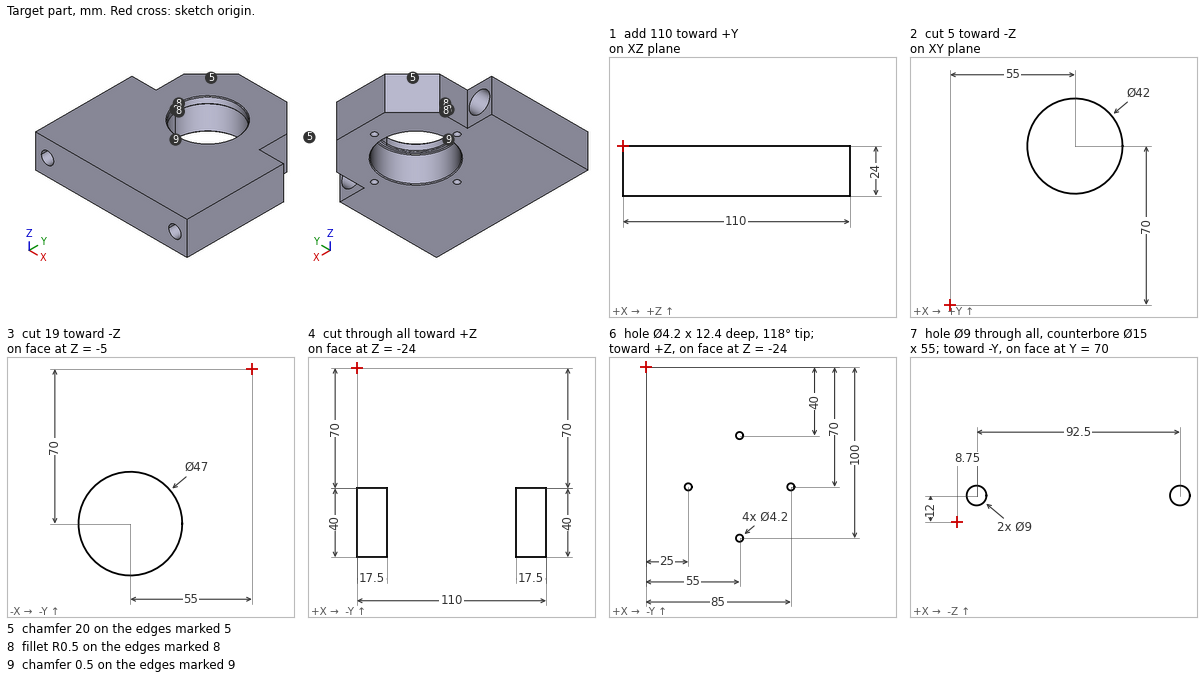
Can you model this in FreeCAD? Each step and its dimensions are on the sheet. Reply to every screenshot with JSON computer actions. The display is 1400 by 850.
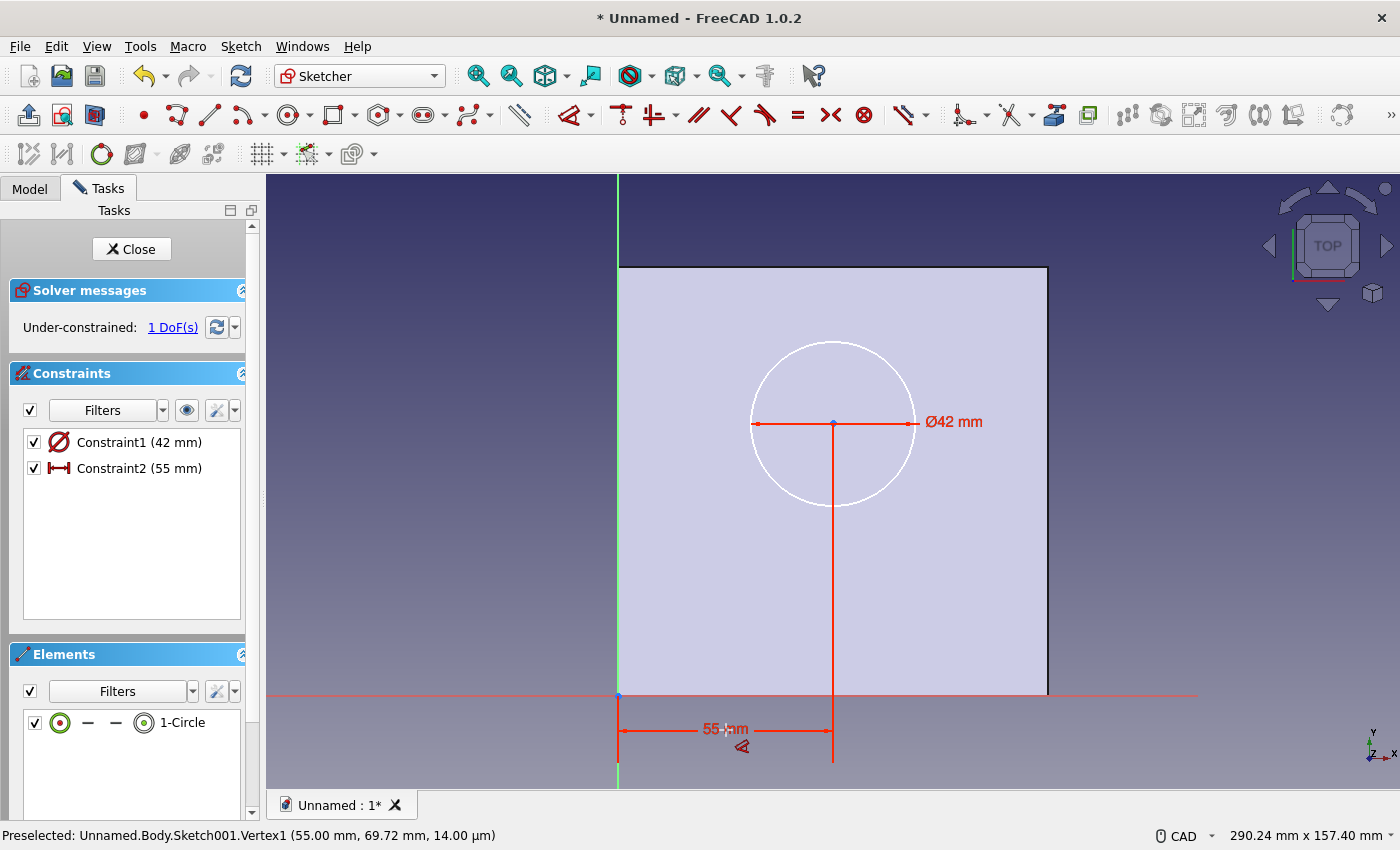
{"action": "left_click", "coordinate": [833, 424]}
{"action": "left_click", "coordinate": [584, 560]}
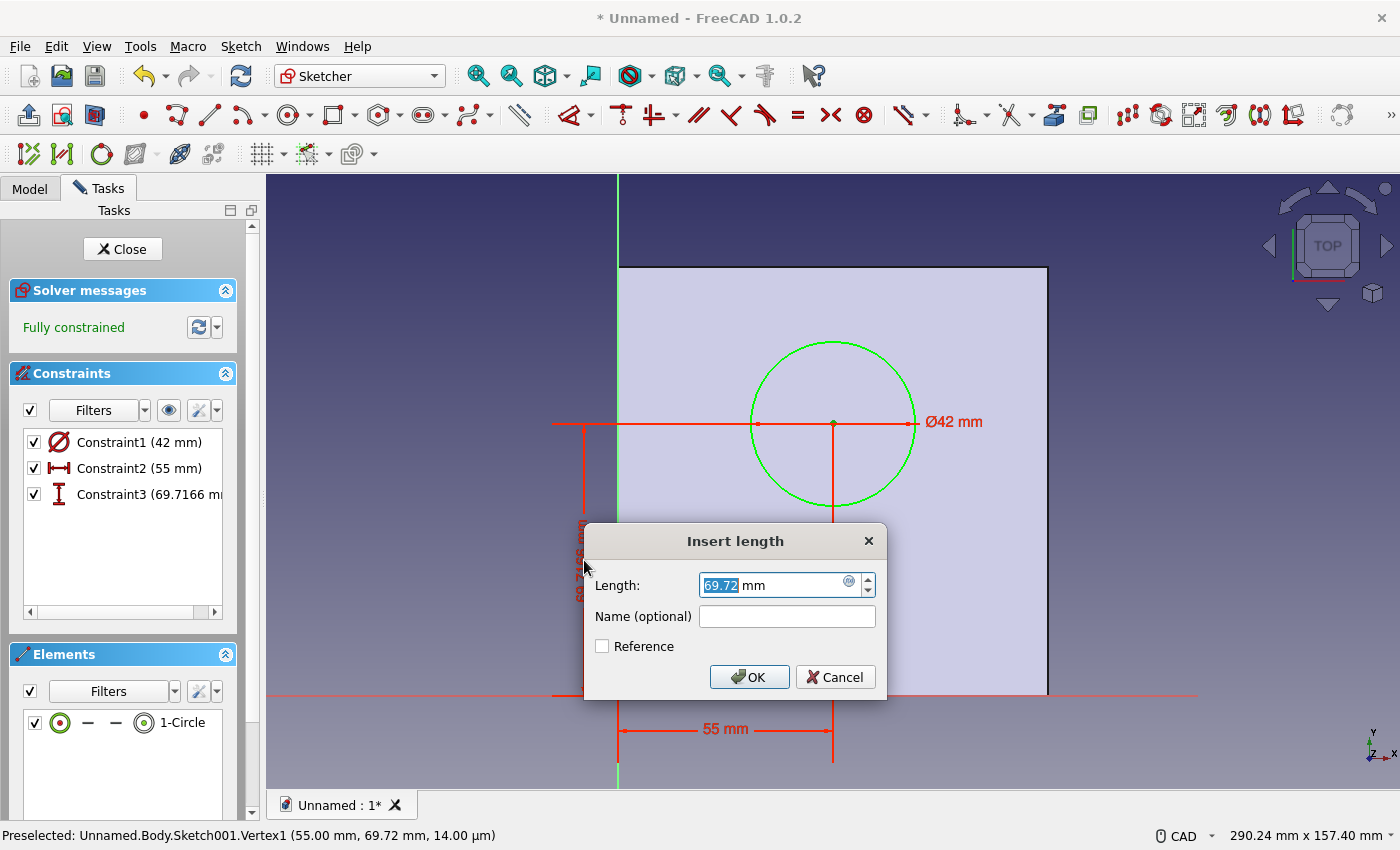
{"action": "type", "text": "70"}
{"action": "key", "text": "Return"}
{"action": "key", "text": "Escape"}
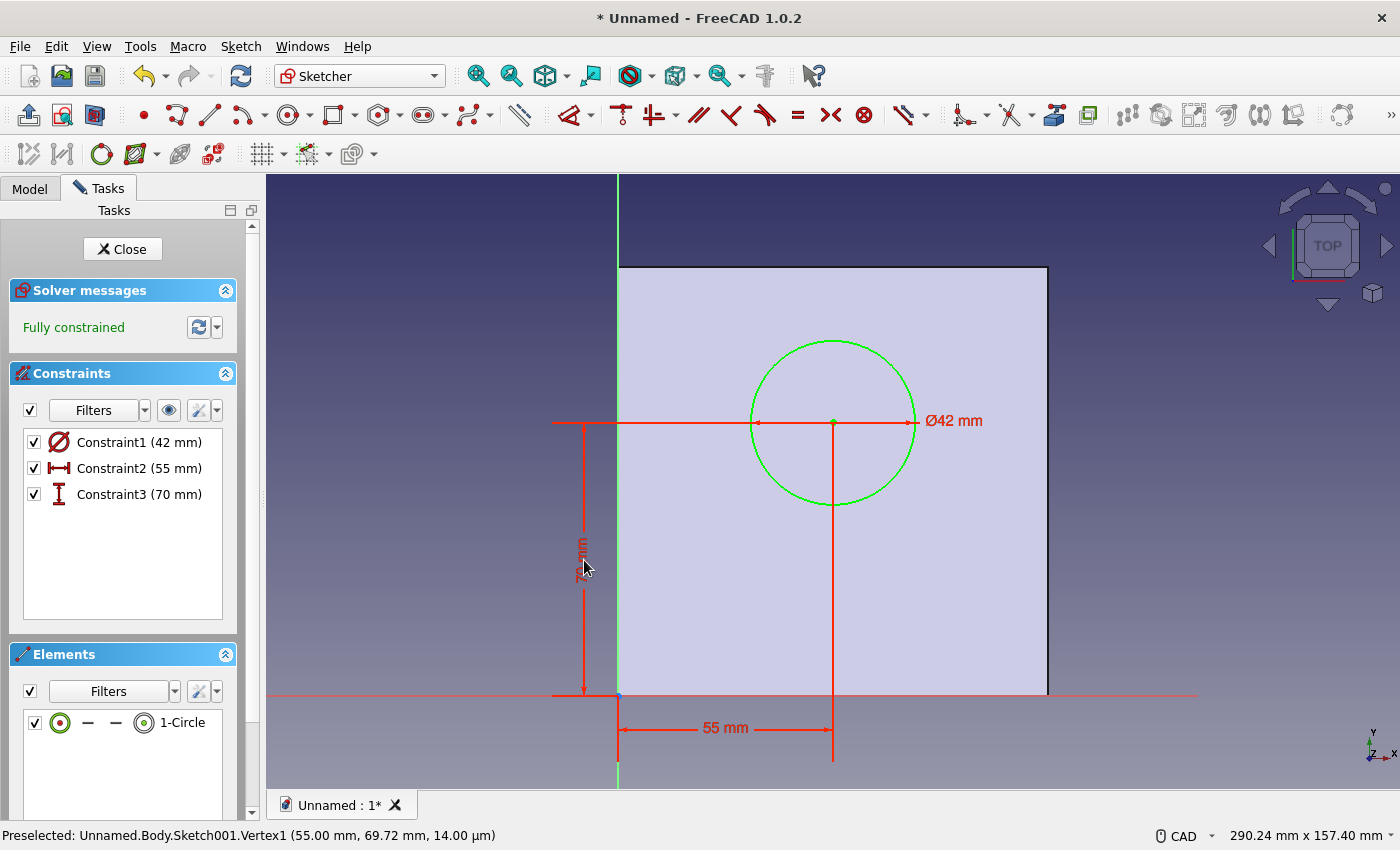
{"action": "left_click", "coordinate": [123, 249]}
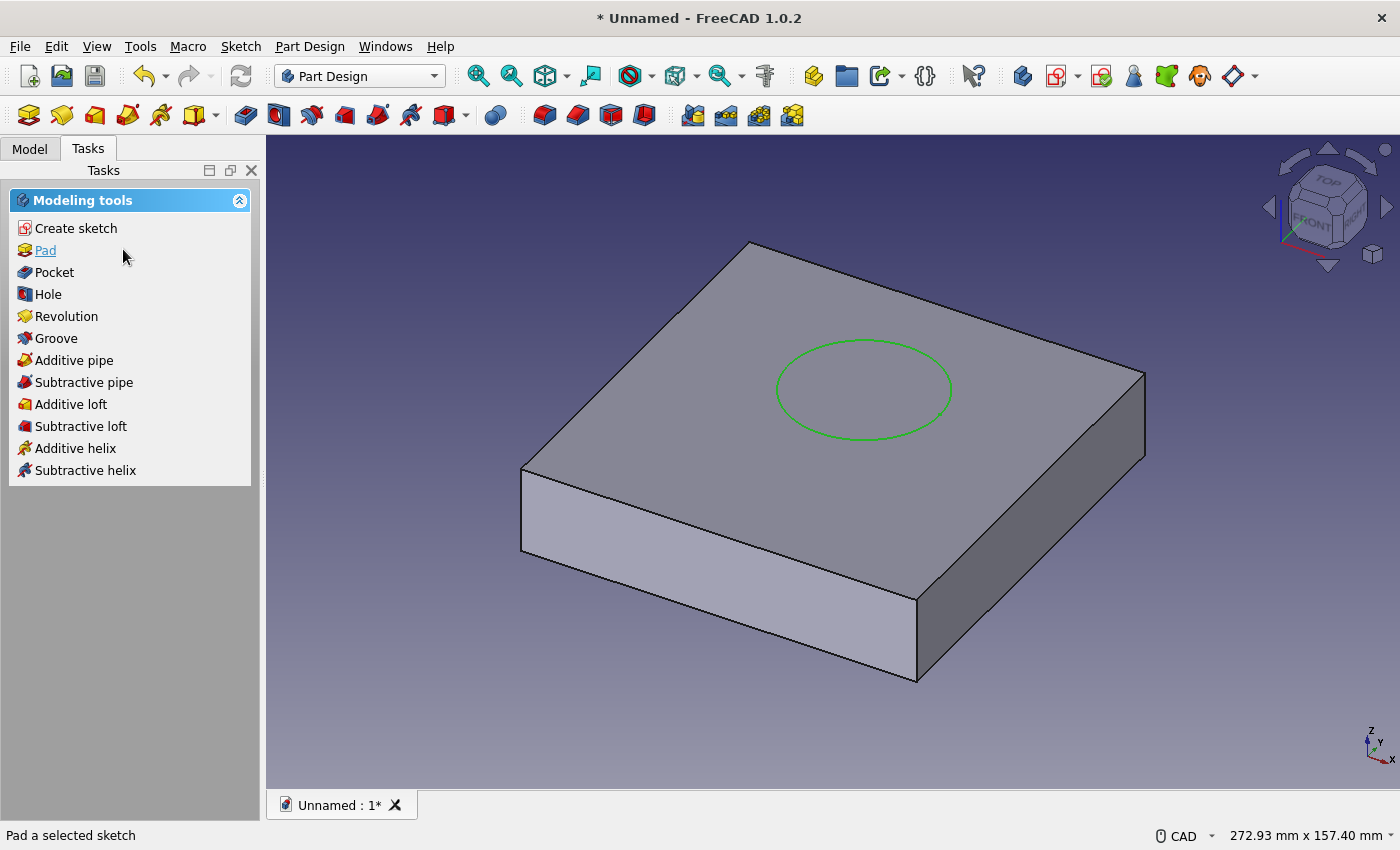
{"action": "left_click", "coordinate": [246, 116]}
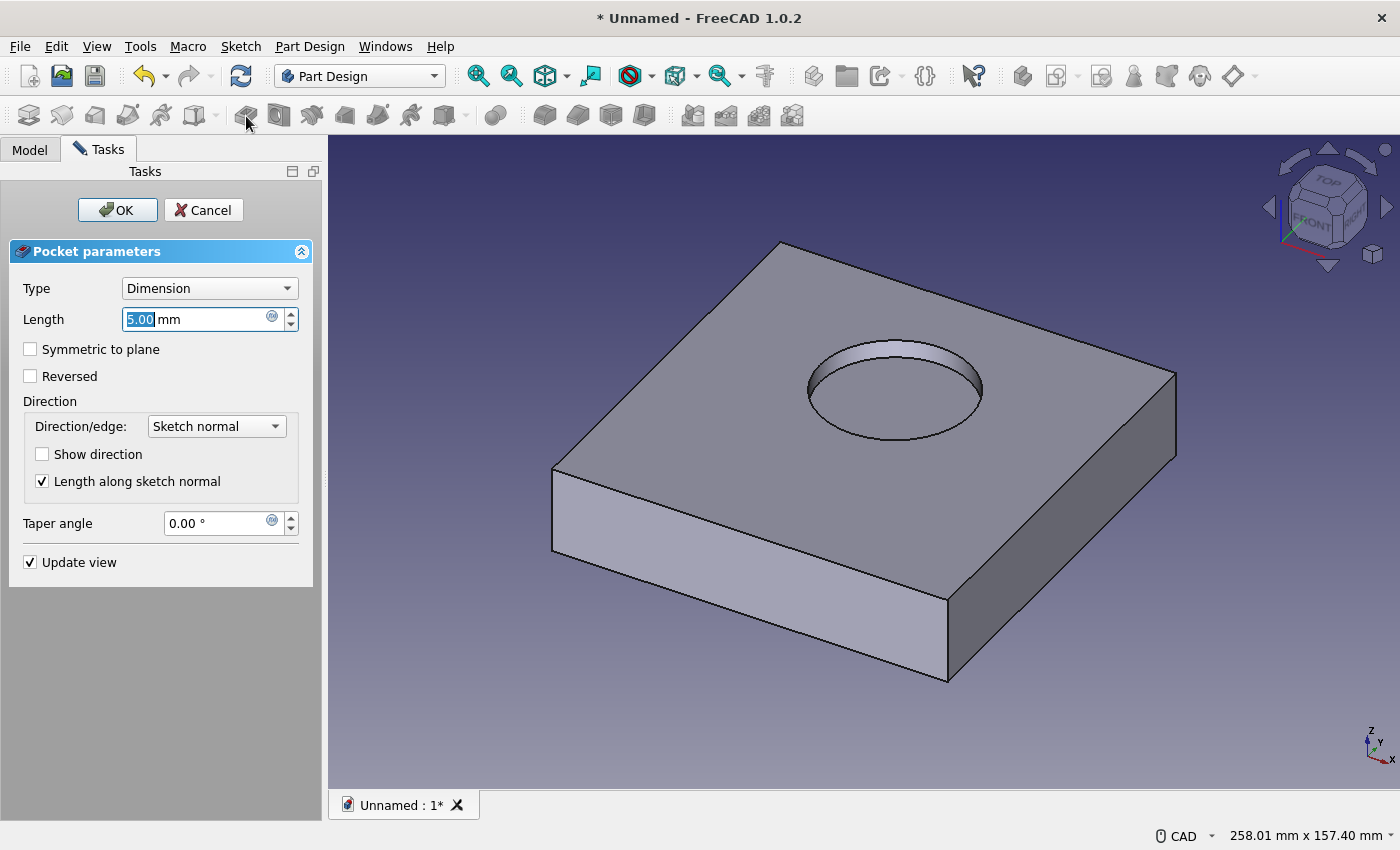
{"action": "type", "text": "5"}
{"action": "key", "text": "Tab"}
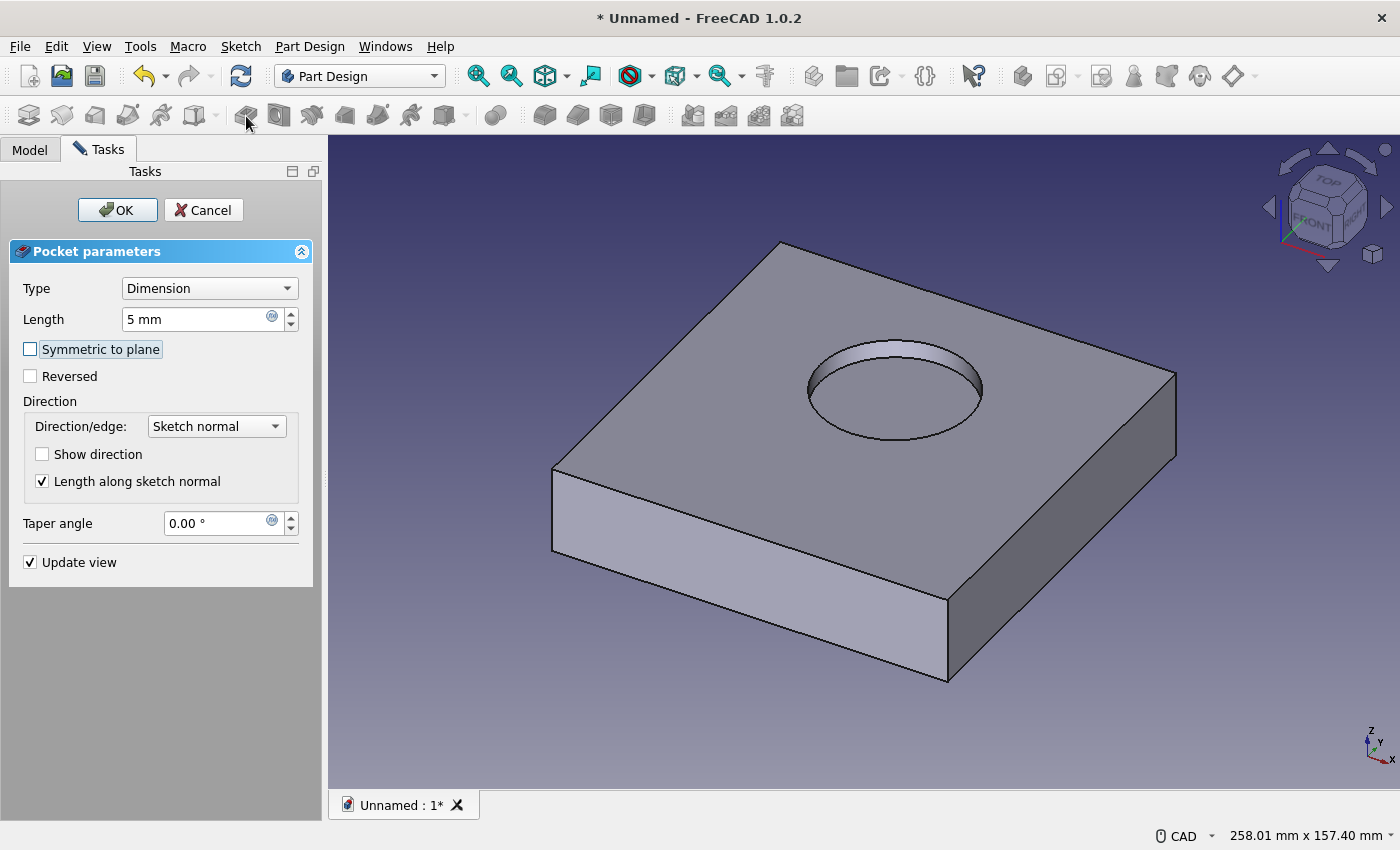
{"action": "left_click", "coordinate": [118, 210]}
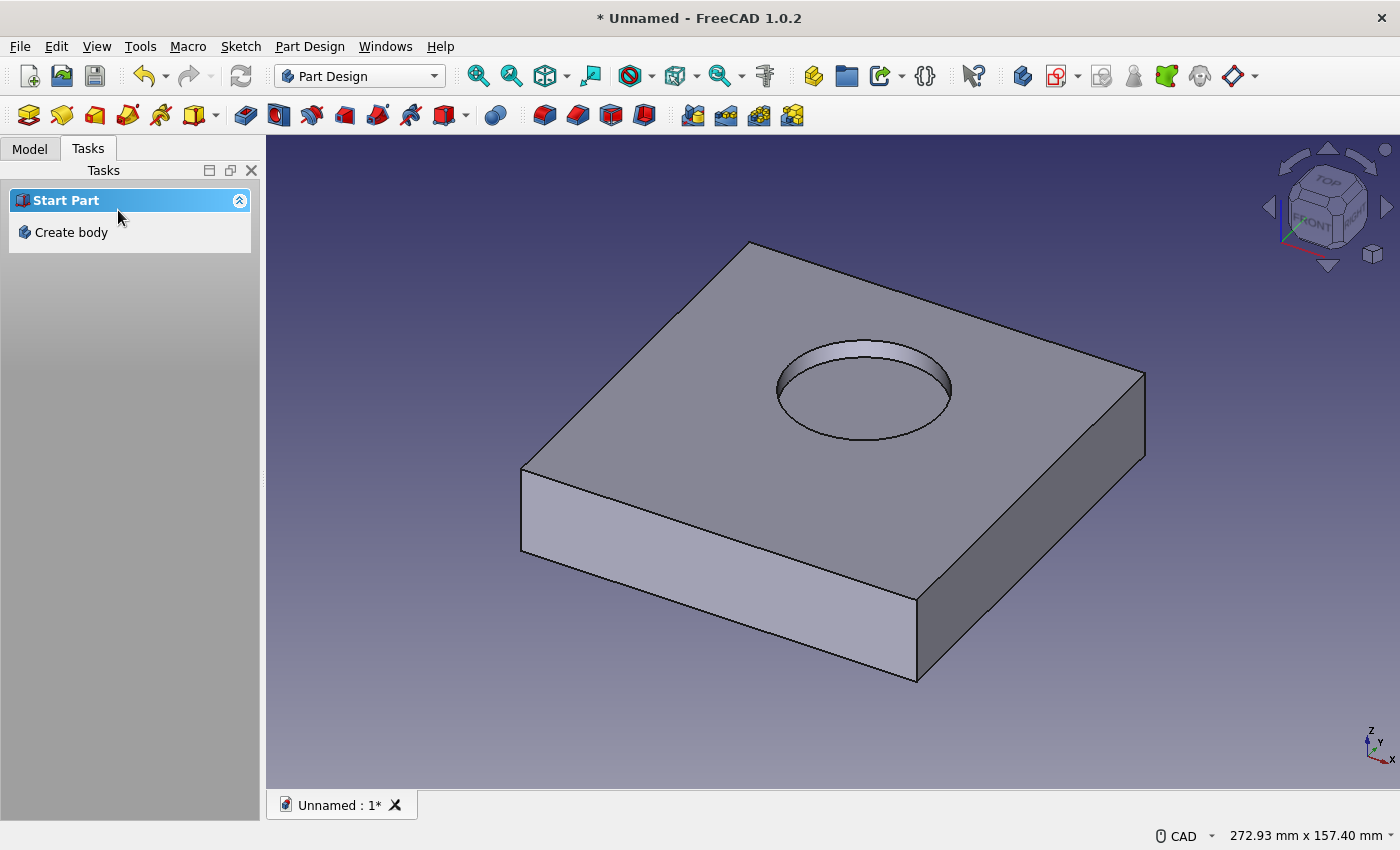
{"action": "left_click", "coordinate": [864, 406]}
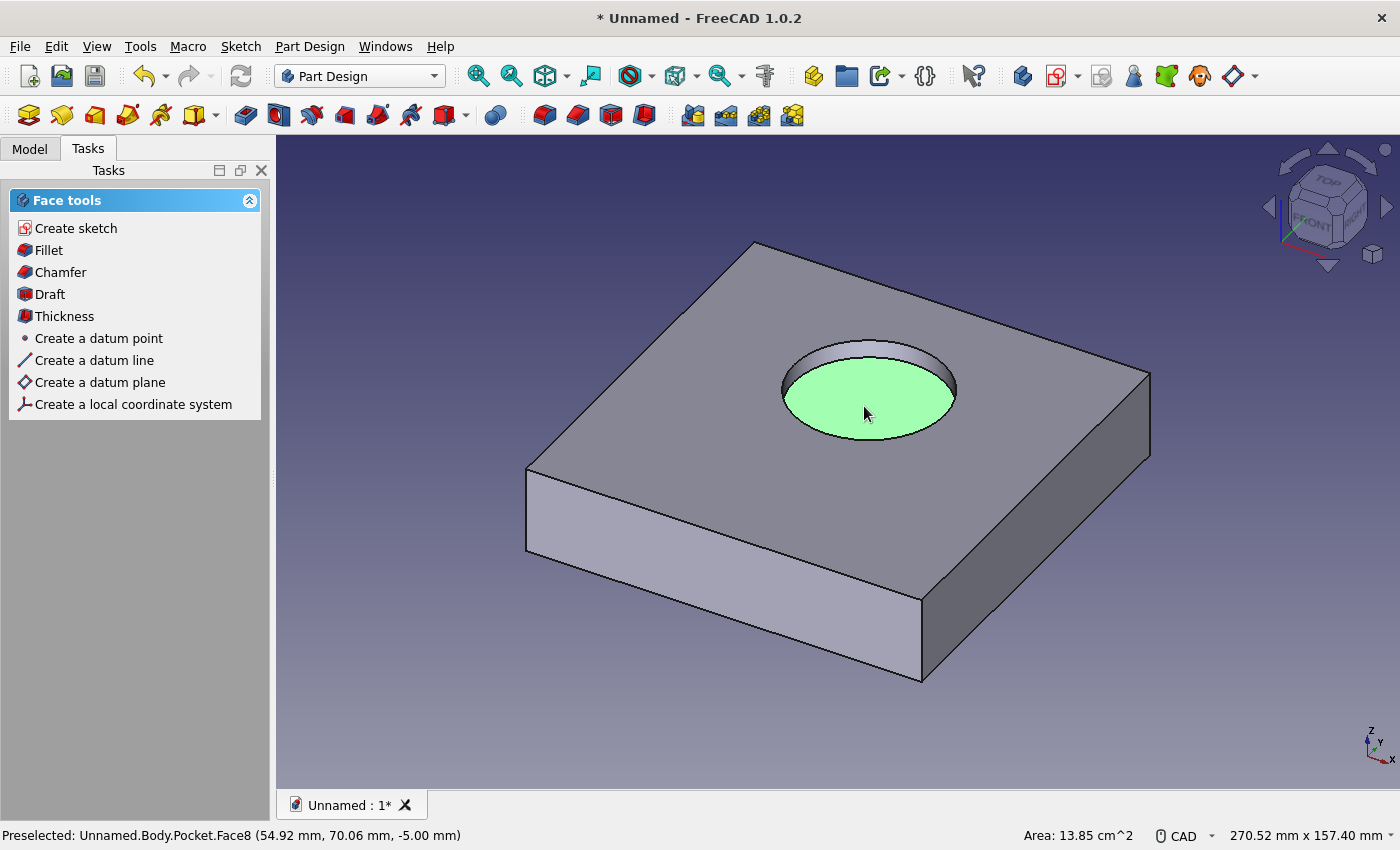
{"action": "left_click", "coordinate": [1056, 76]}